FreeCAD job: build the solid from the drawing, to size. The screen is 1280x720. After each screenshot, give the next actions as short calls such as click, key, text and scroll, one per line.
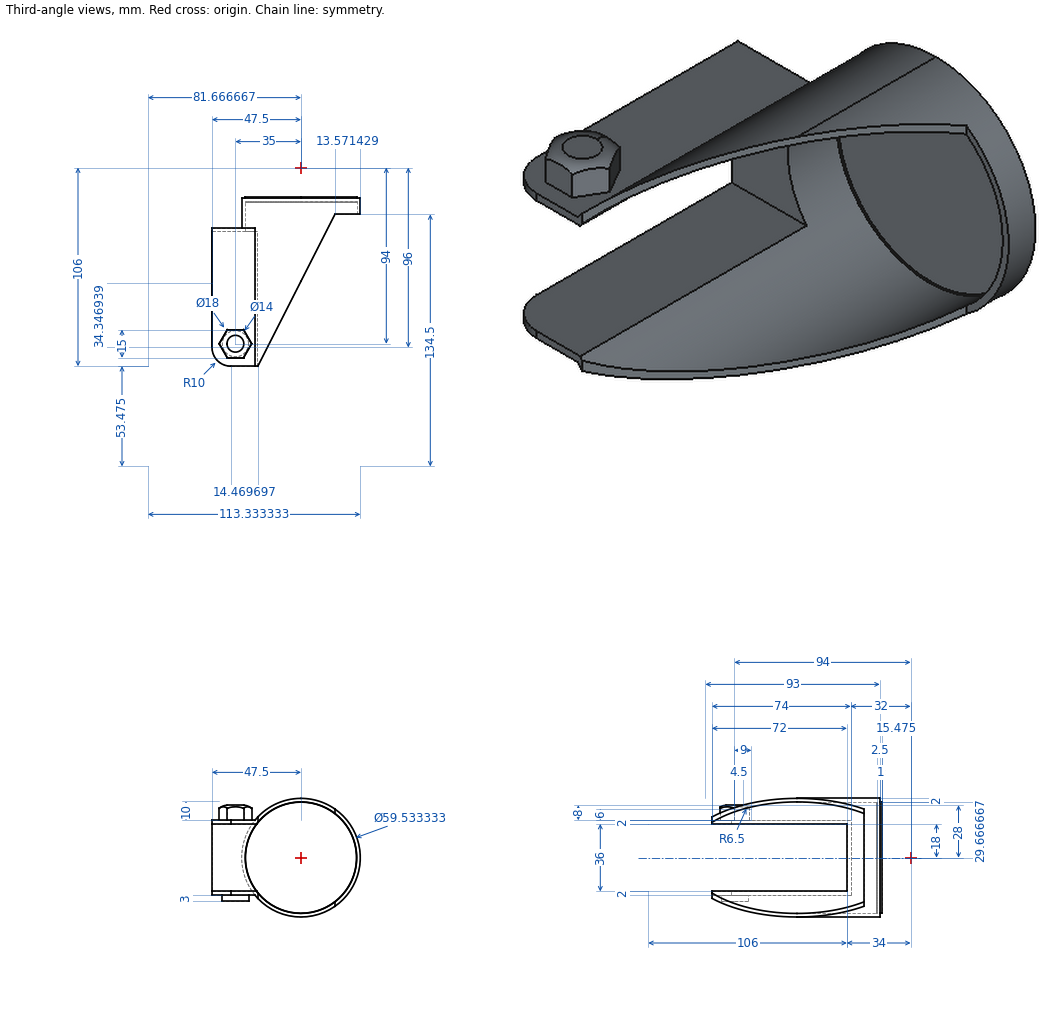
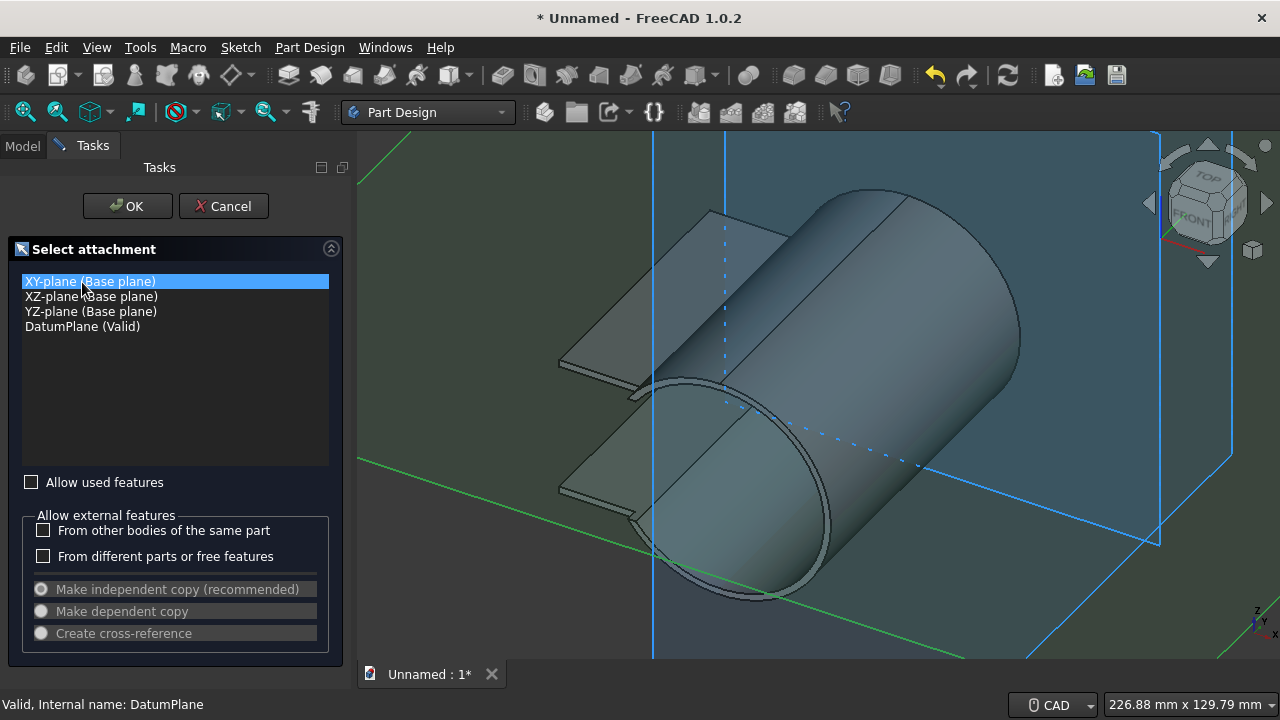
click(128, 206)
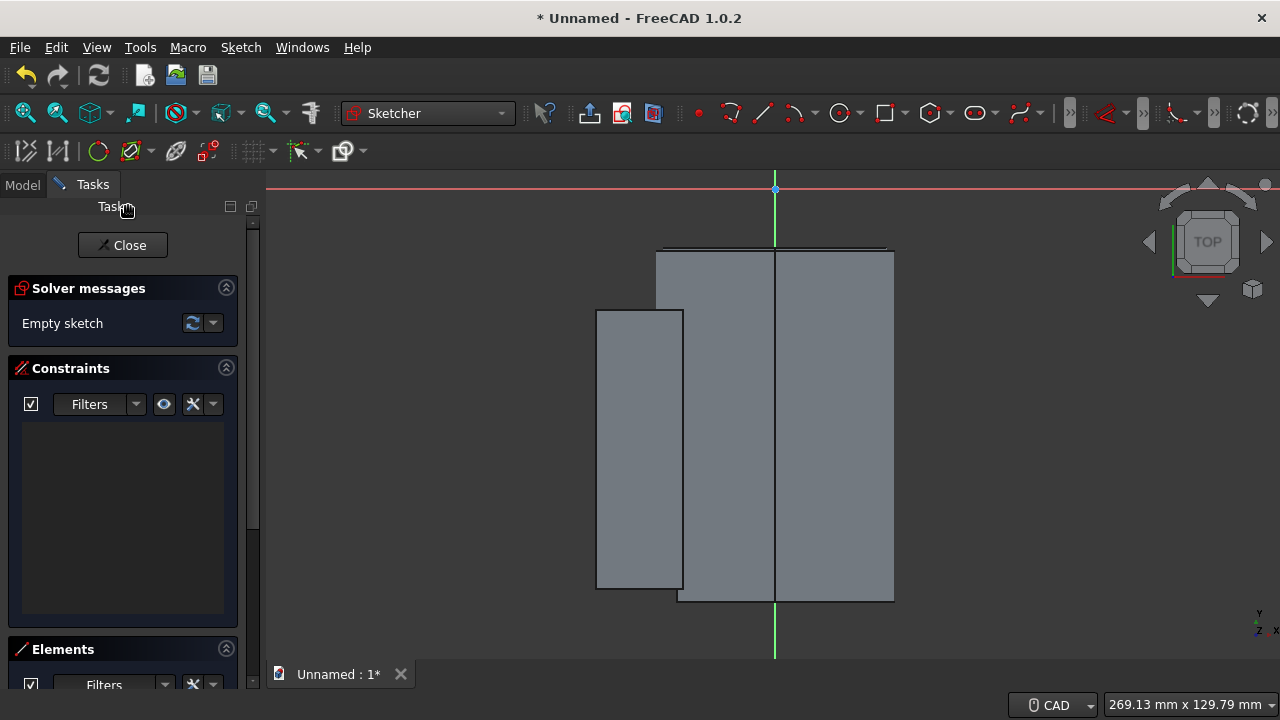
key(q)
key(s)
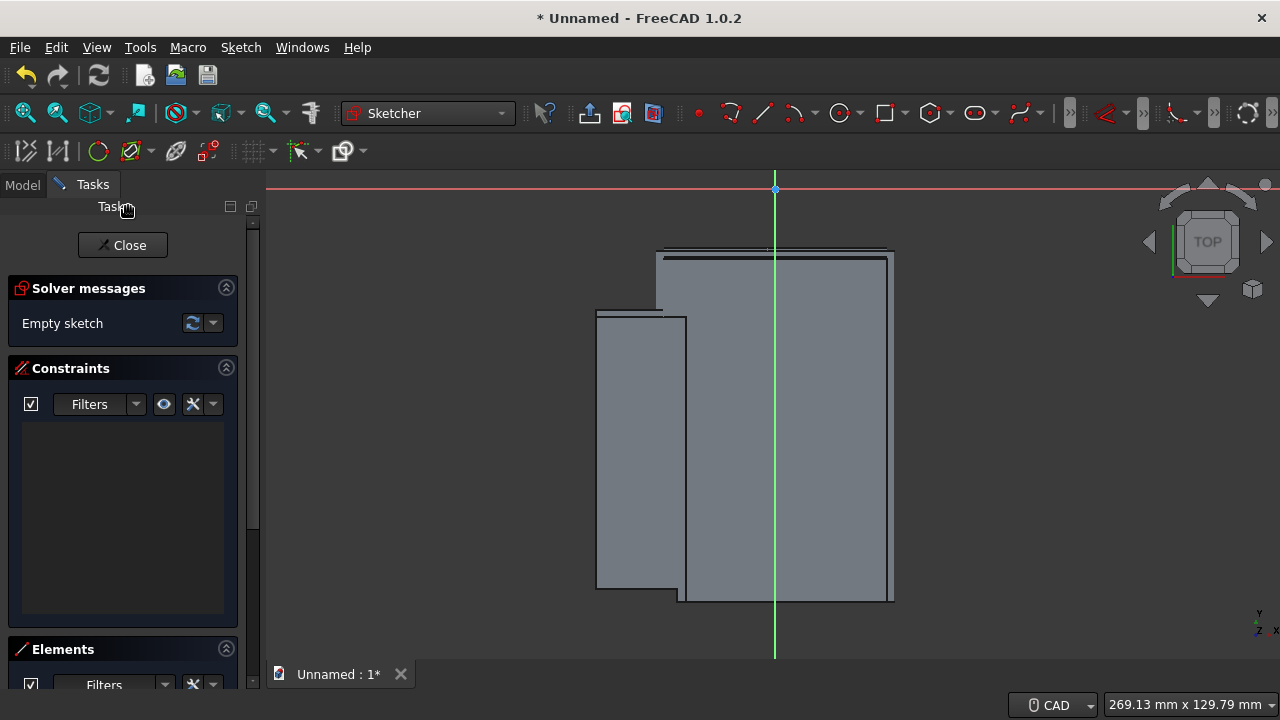
scroll(733, 323, down, 3)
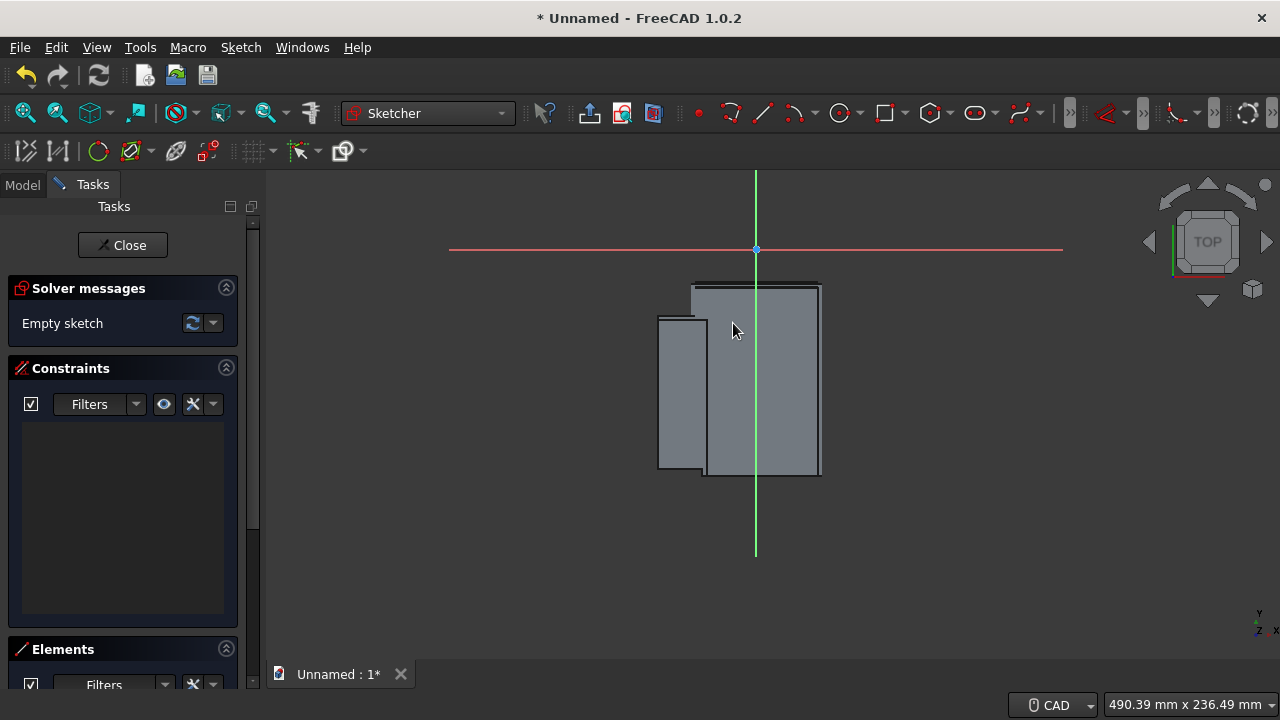
key(g)
key(m)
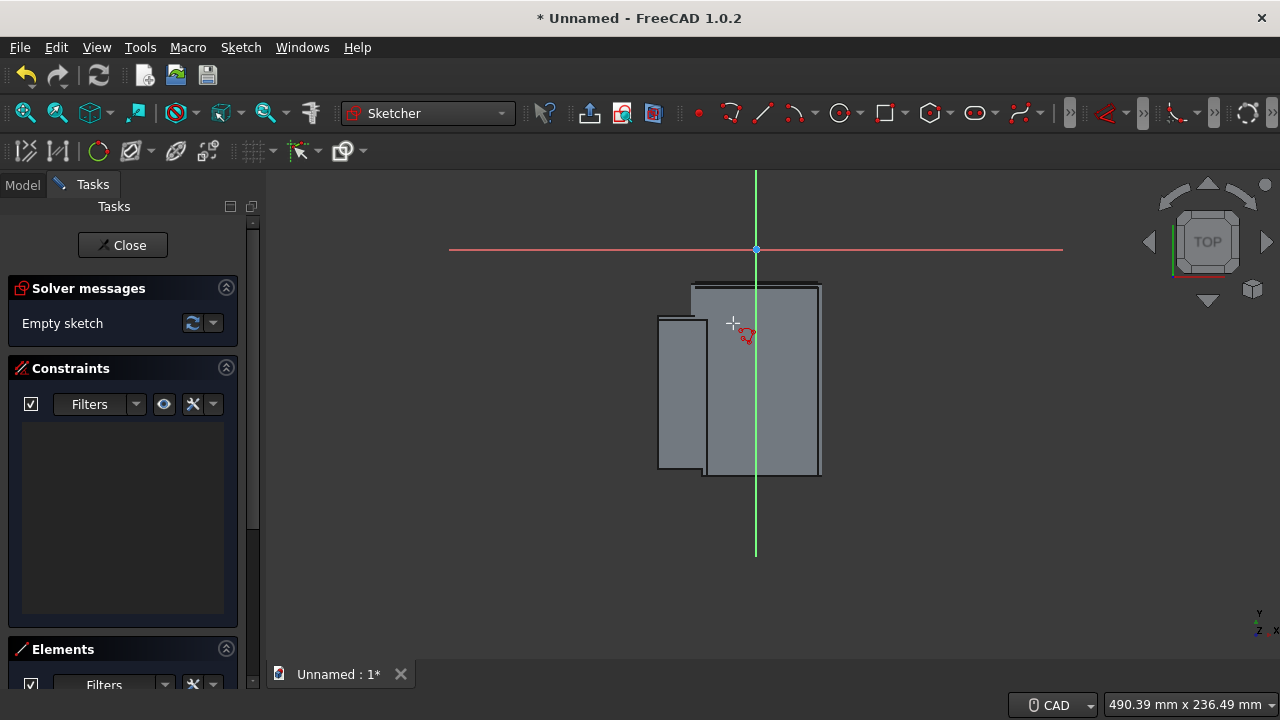
click(658, 448)
click(658, 377)
click(587, 469)
click(587, 579)
click(822, 579)
click(822, 301)
click(794, 301)
click(709, 469)
click(679, 469)
right_click(679, 469)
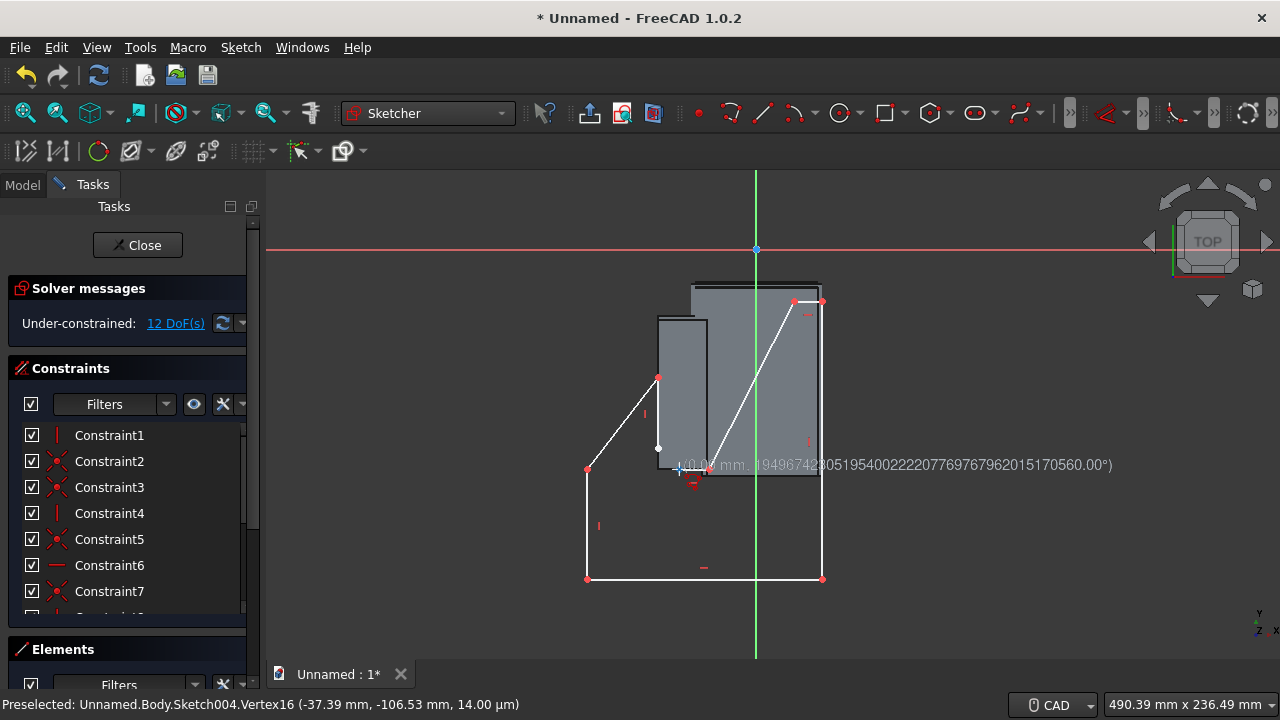
click(818, 114)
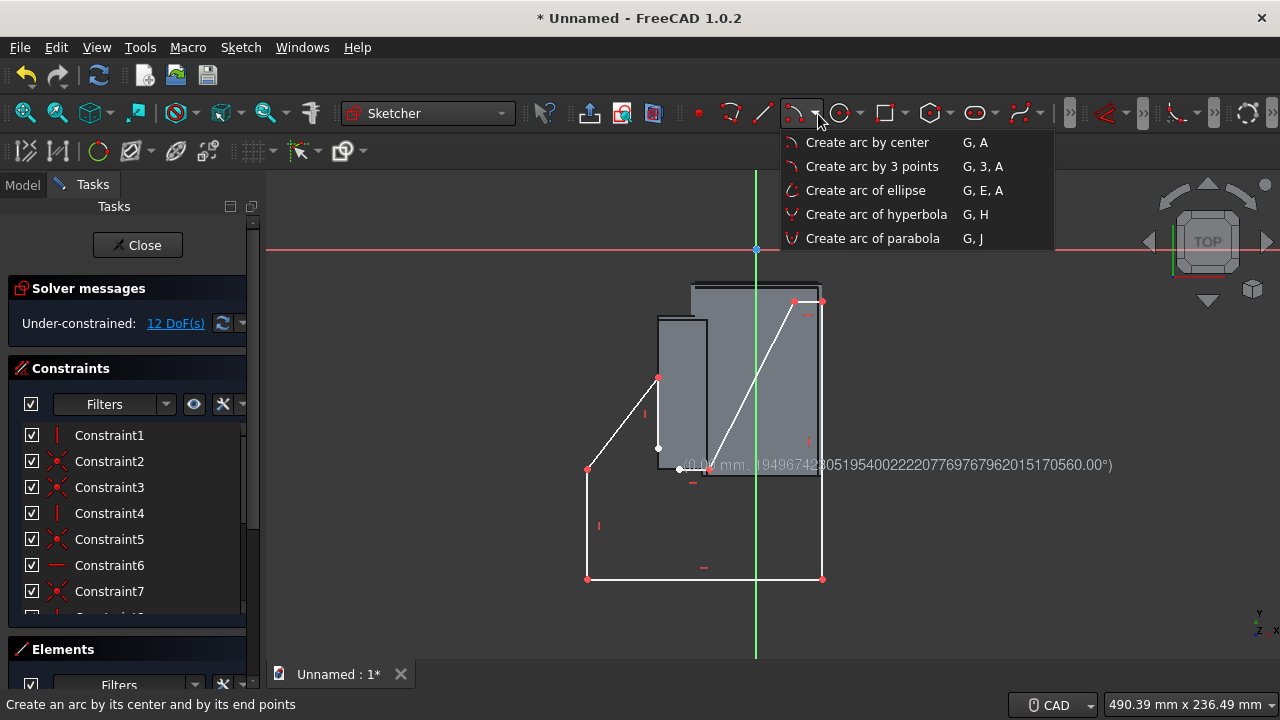
click(918, 166)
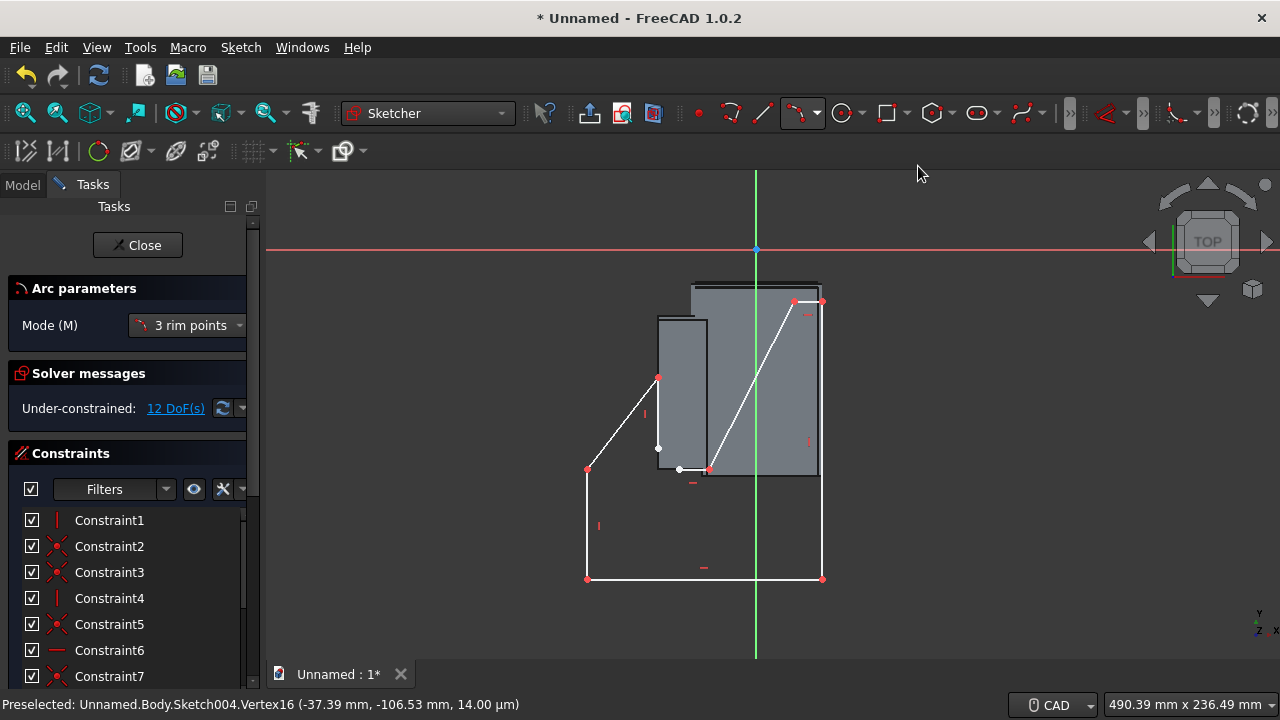
click(679, 470)
click(658, 449)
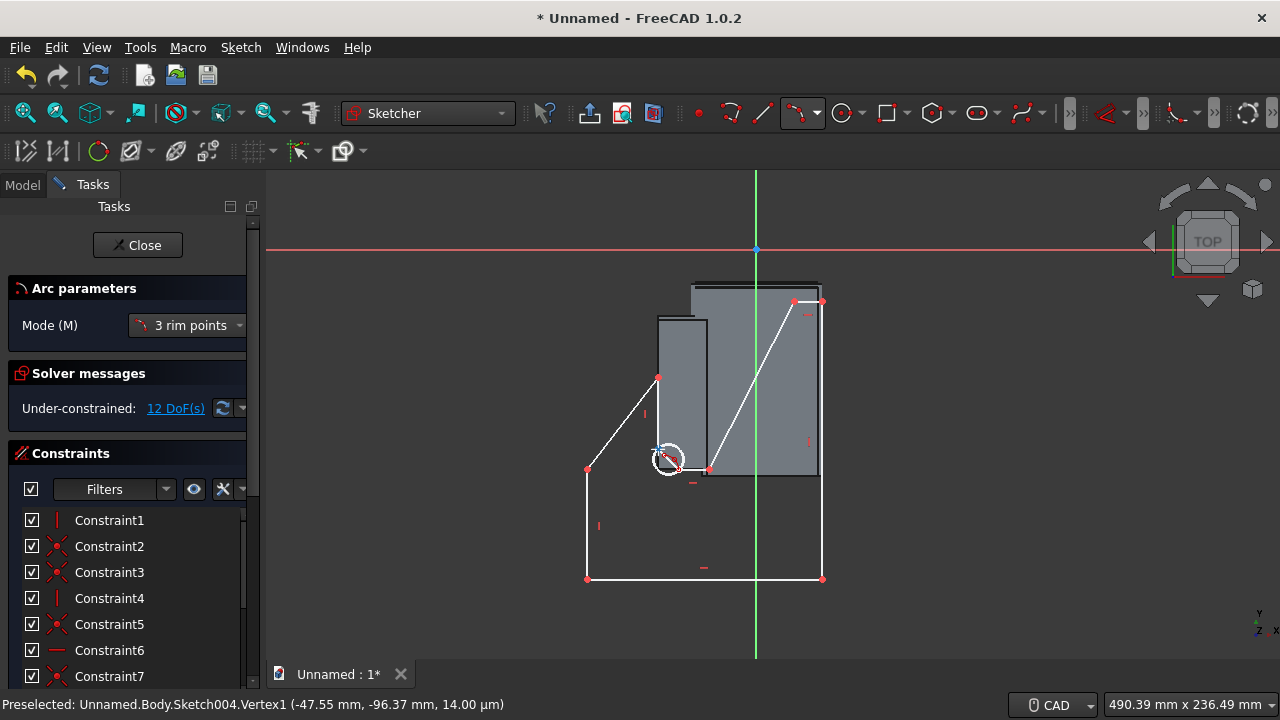
scroll(664, 463, up, 5)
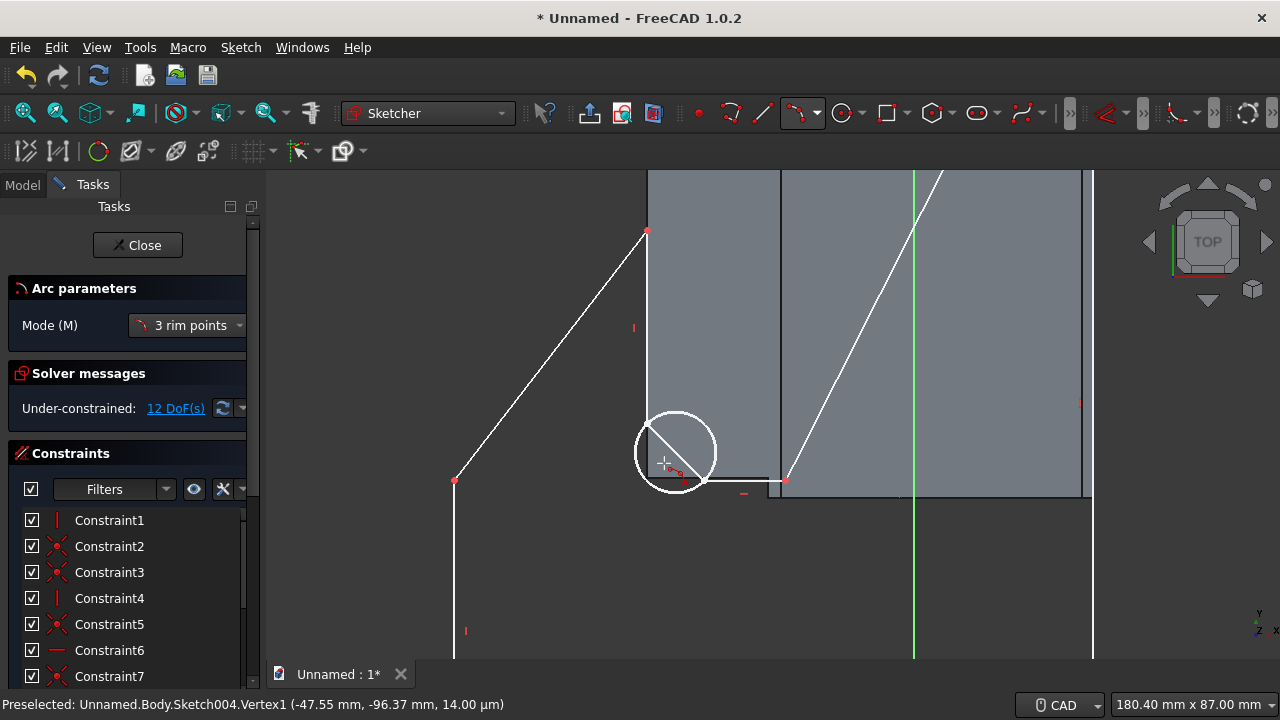
click(664, 462)
key(Escape)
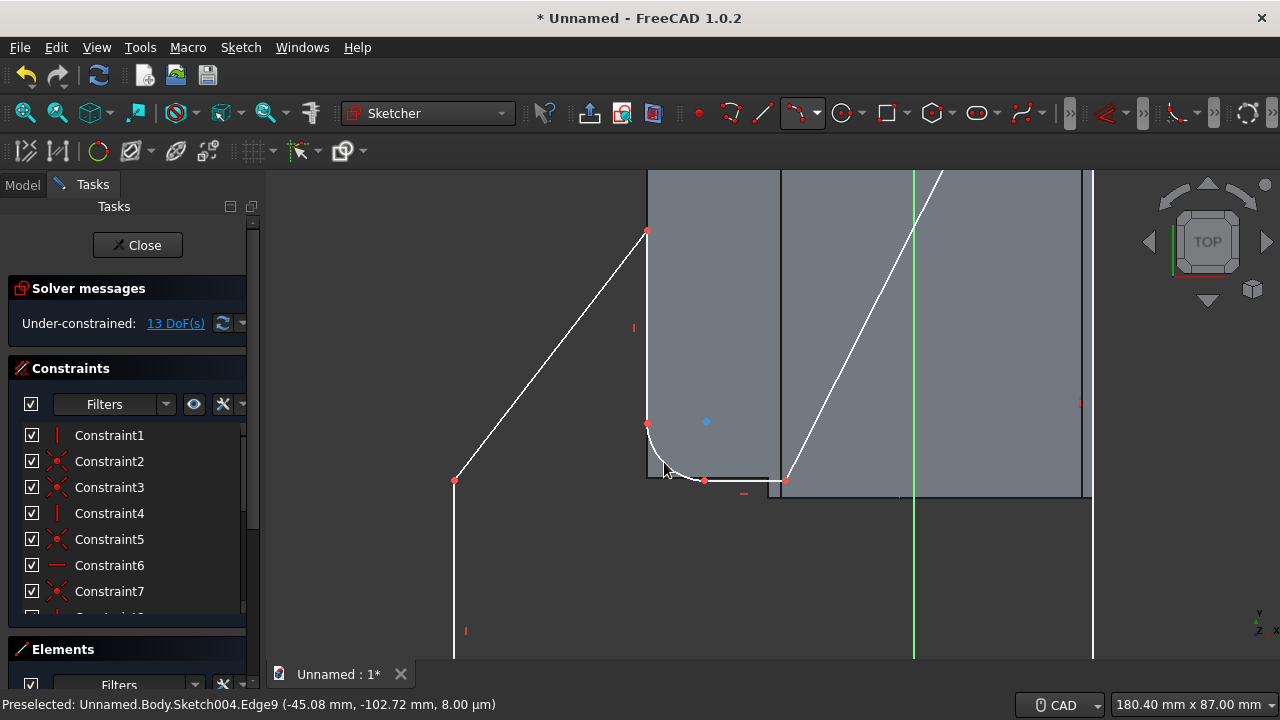
click(647, 366)